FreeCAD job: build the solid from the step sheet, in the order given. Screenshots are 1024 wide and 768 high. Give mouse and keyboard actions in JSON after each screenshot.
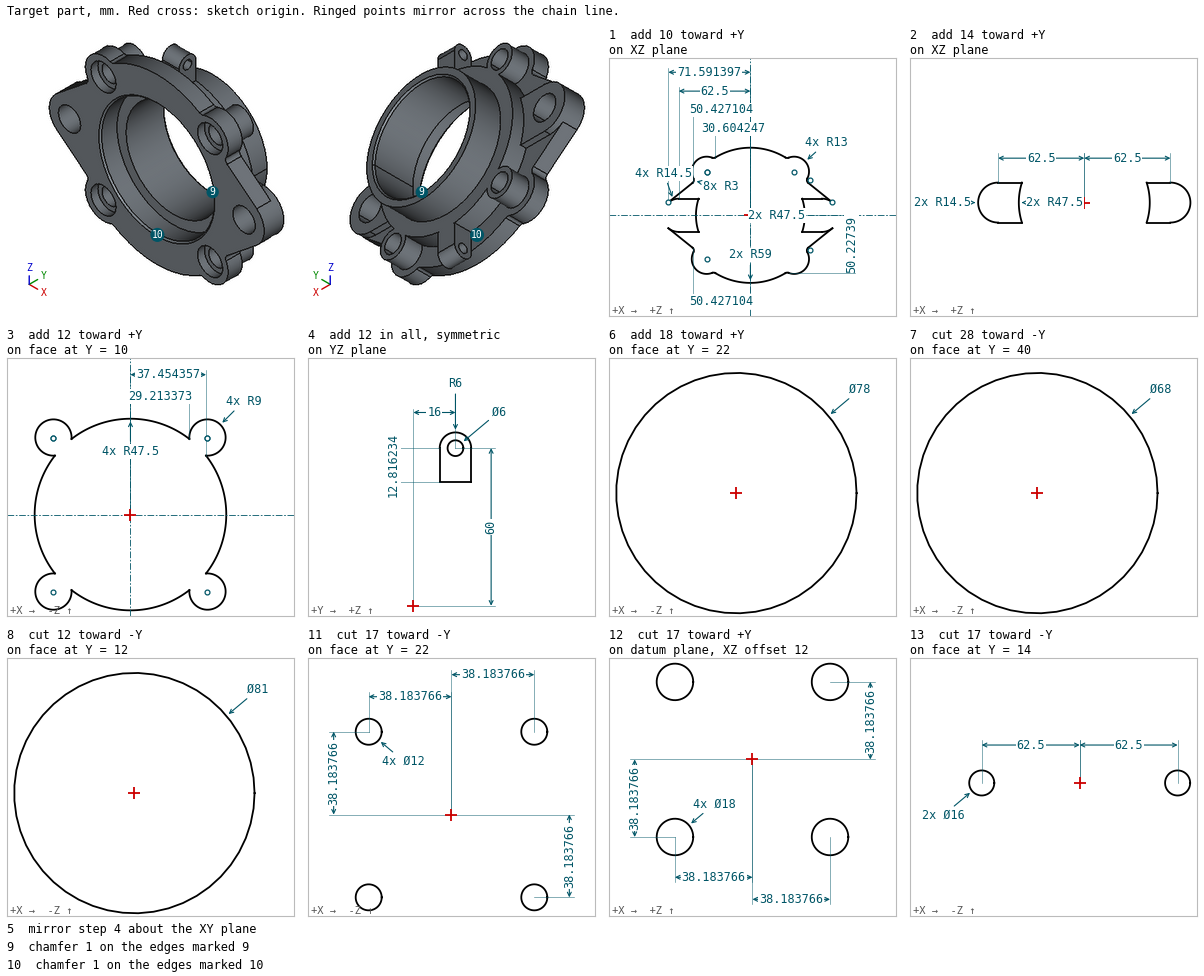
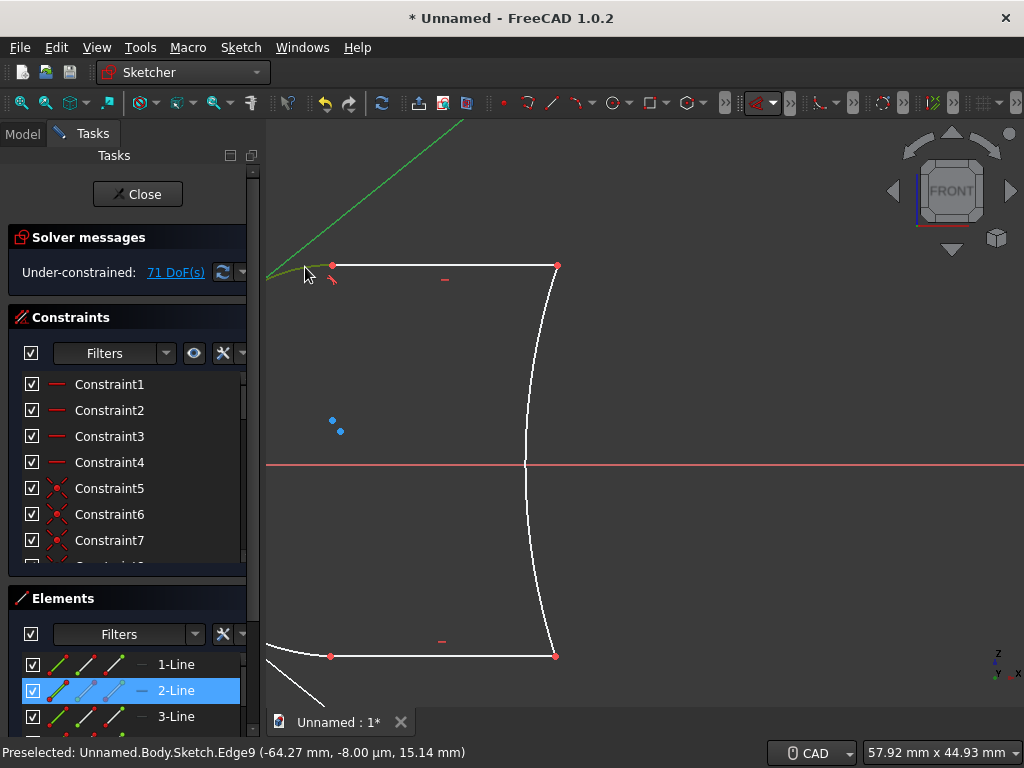
{"action": "key", "text": "t"}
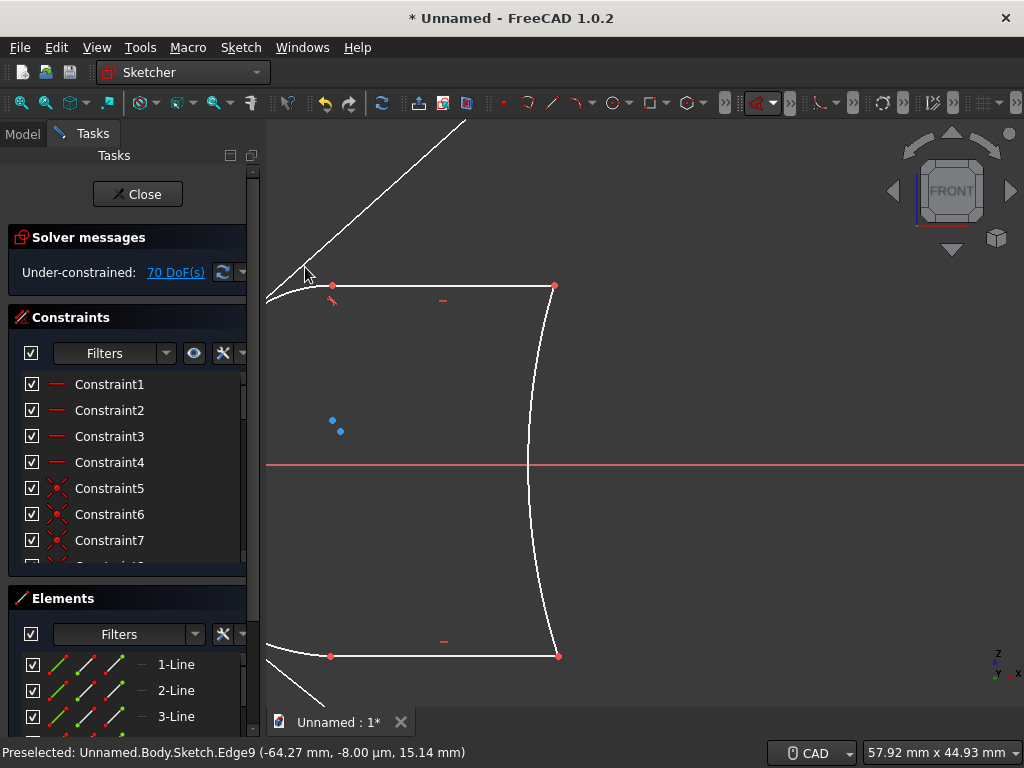
{"action": "left_click", "coordinate": [316, 253]}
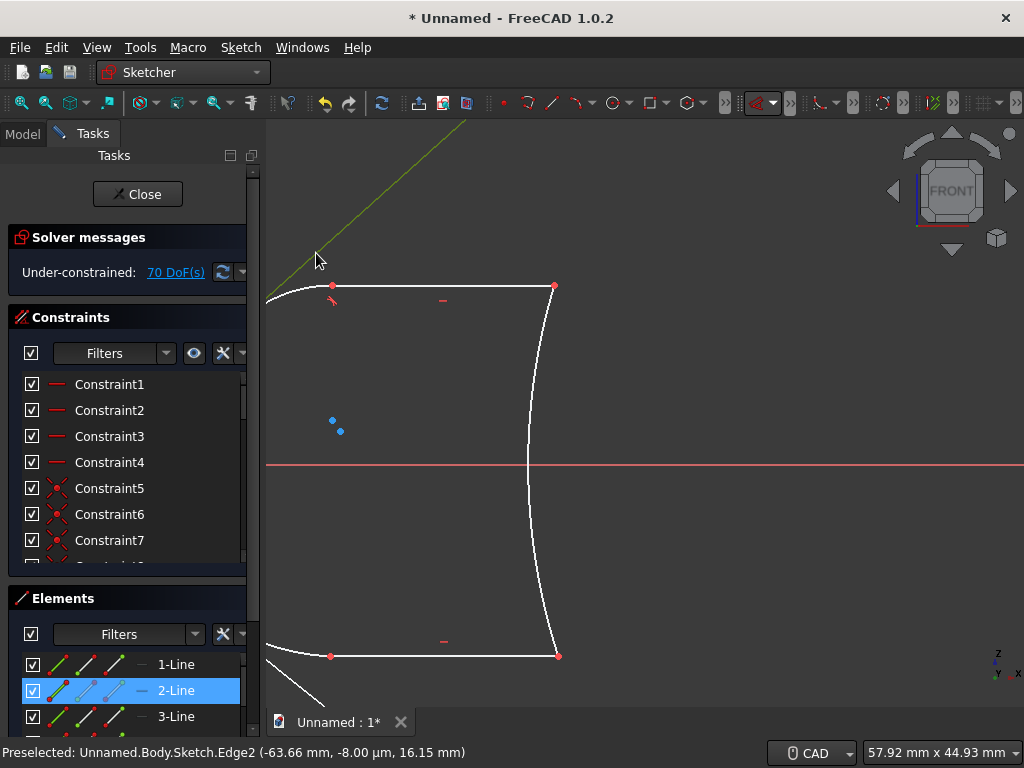
{"action": "scroll", "coordinate": [432, 400], "scroll_direction": "down", "scroll_amount": 8}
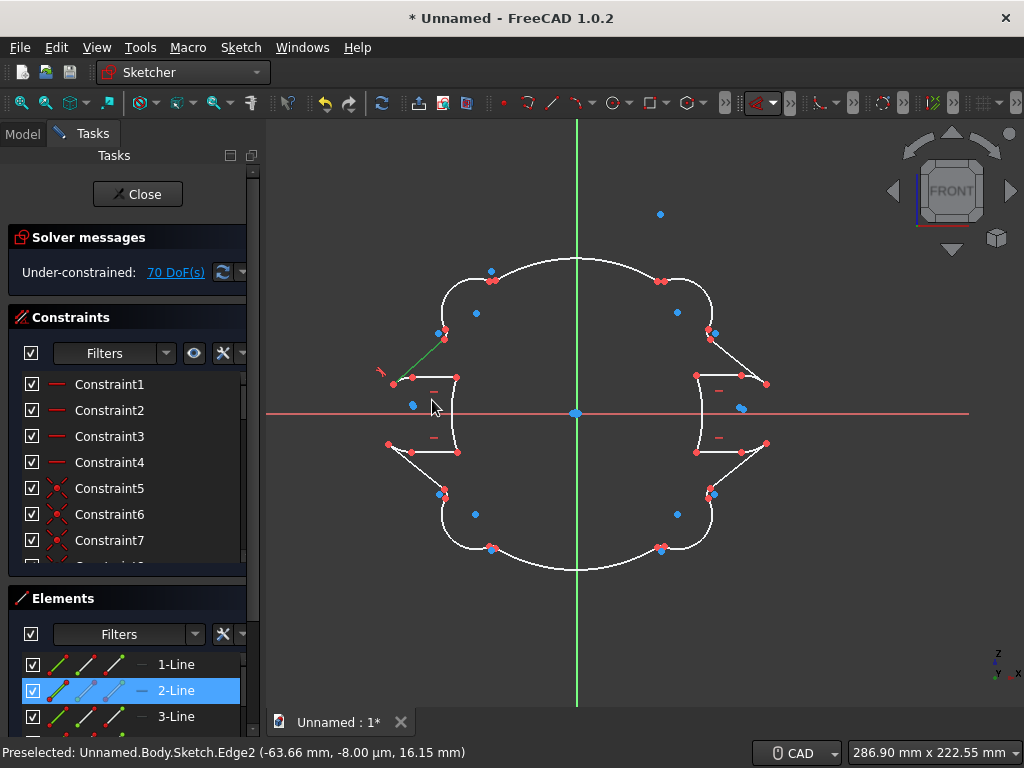
{"action": "scroll", "coordinate": [446, 337], "scroll_direction": "up", "scroll_amount": 8}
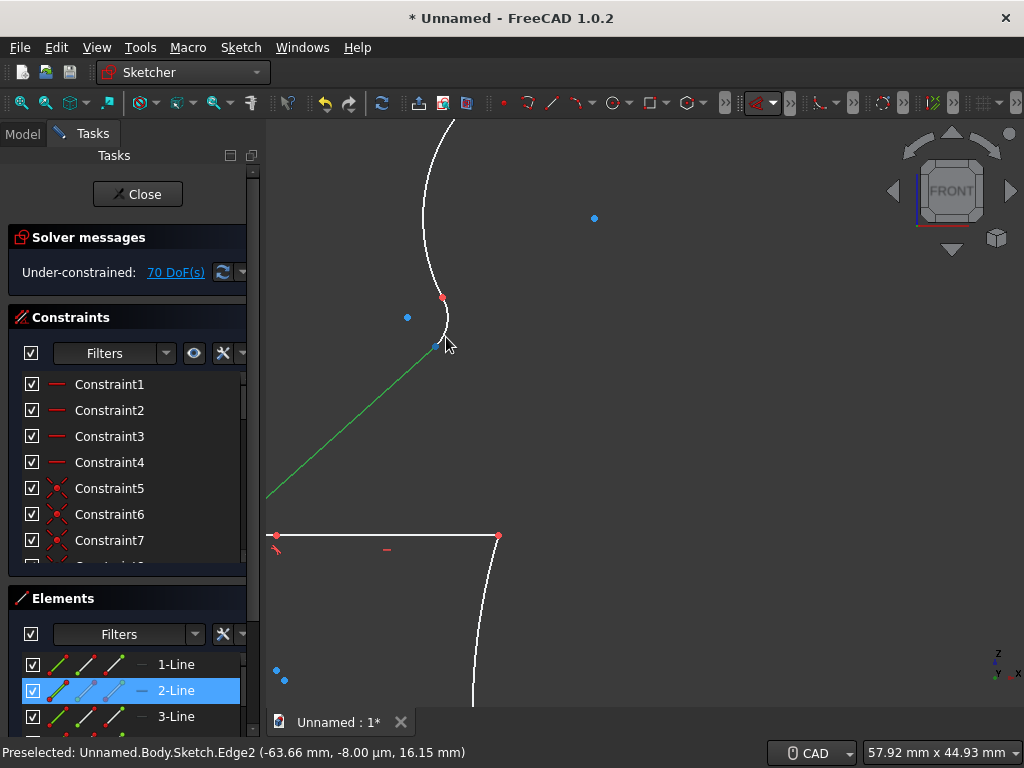
{"action": "left_click", "coordinate": [444, 334]}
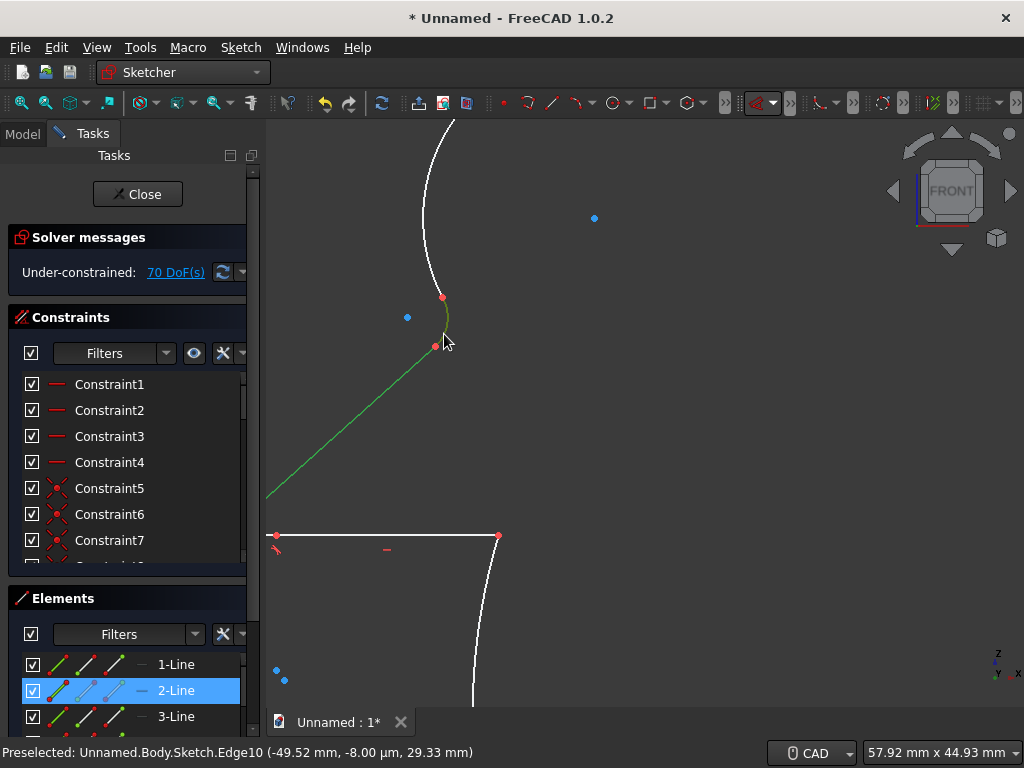
{"action": "key", "text": "t"}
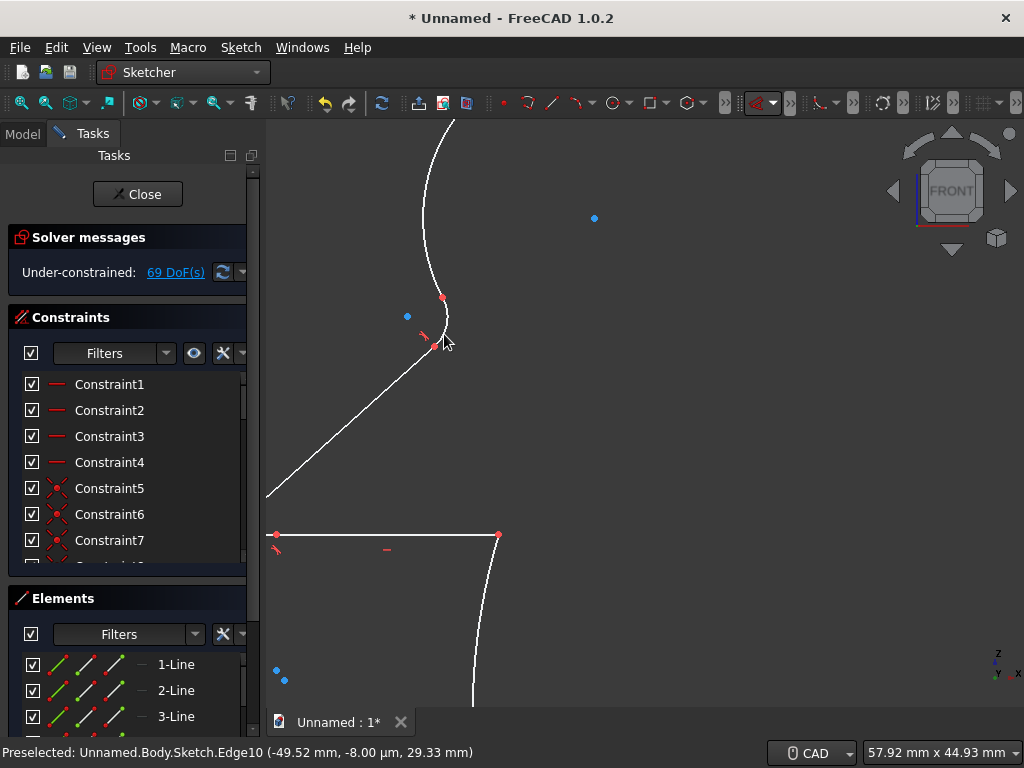
{"action": "scroll", "coordinate": [446, 337], "scroll_direction": "down", "scroll_amount": 8}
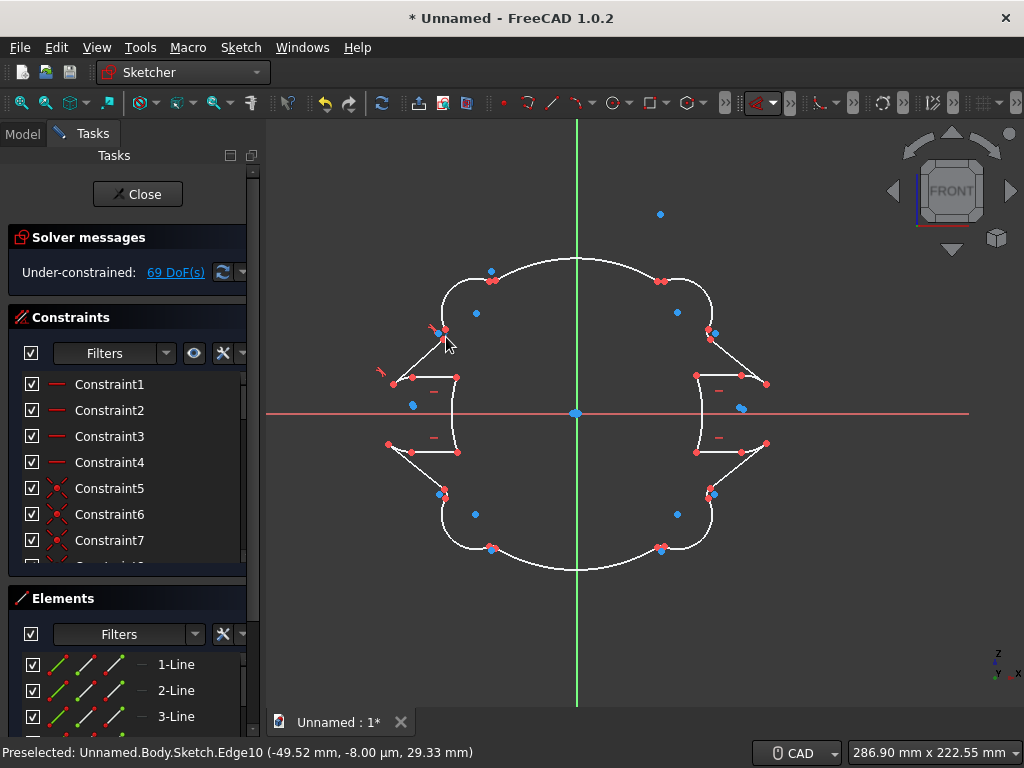
{"action": "left_click", "coordinate": [727, 353]}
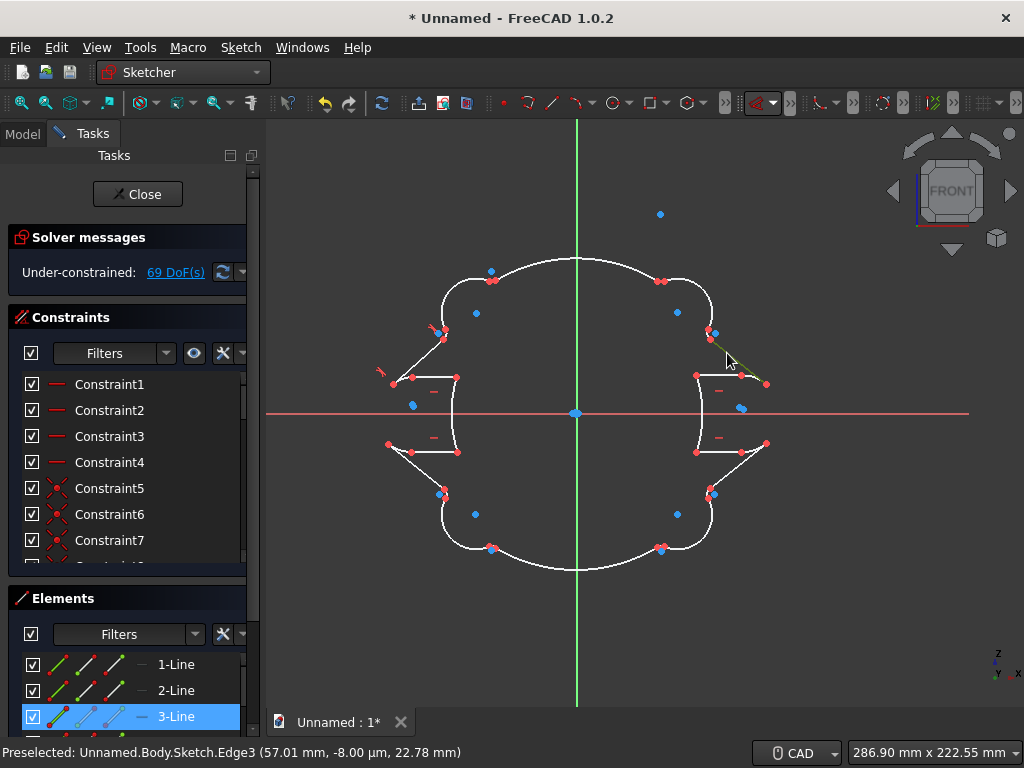
{"action": "scroll", "coordinate": [707, 334], "scroll_direction": "up", "scroll_amount": 5}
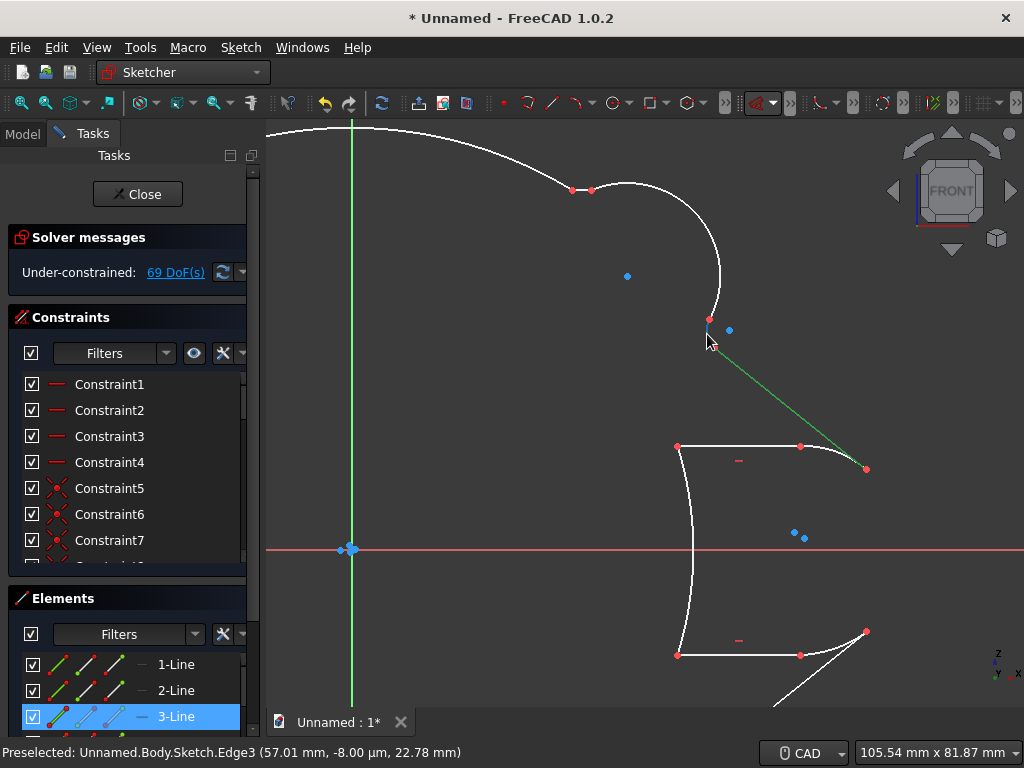
{"action": "left_click", "coordinate": [707, 335]}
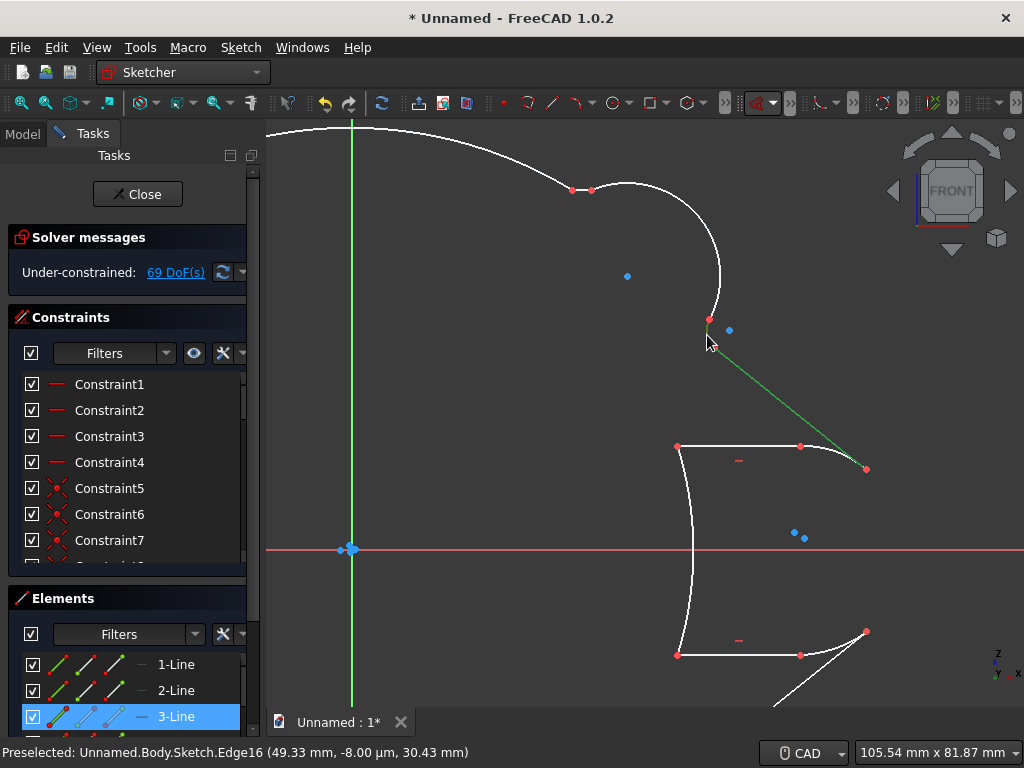
{"action": "key", "text": "t"}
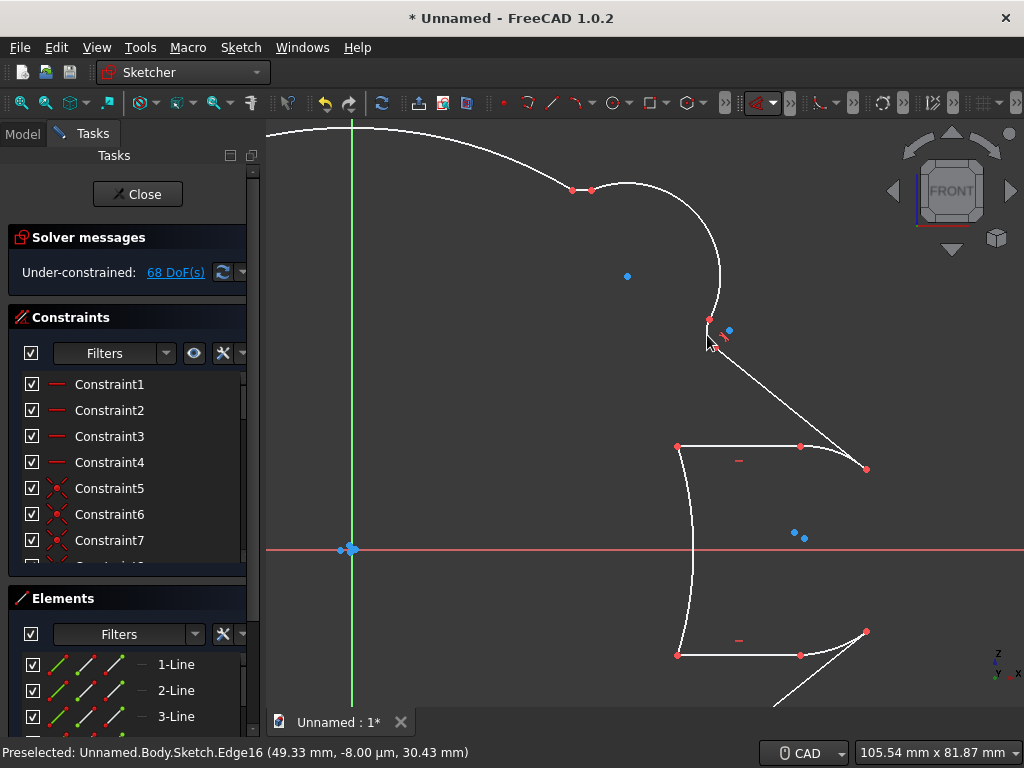
{"action": "left_click", "coordinate": [761, 384]}